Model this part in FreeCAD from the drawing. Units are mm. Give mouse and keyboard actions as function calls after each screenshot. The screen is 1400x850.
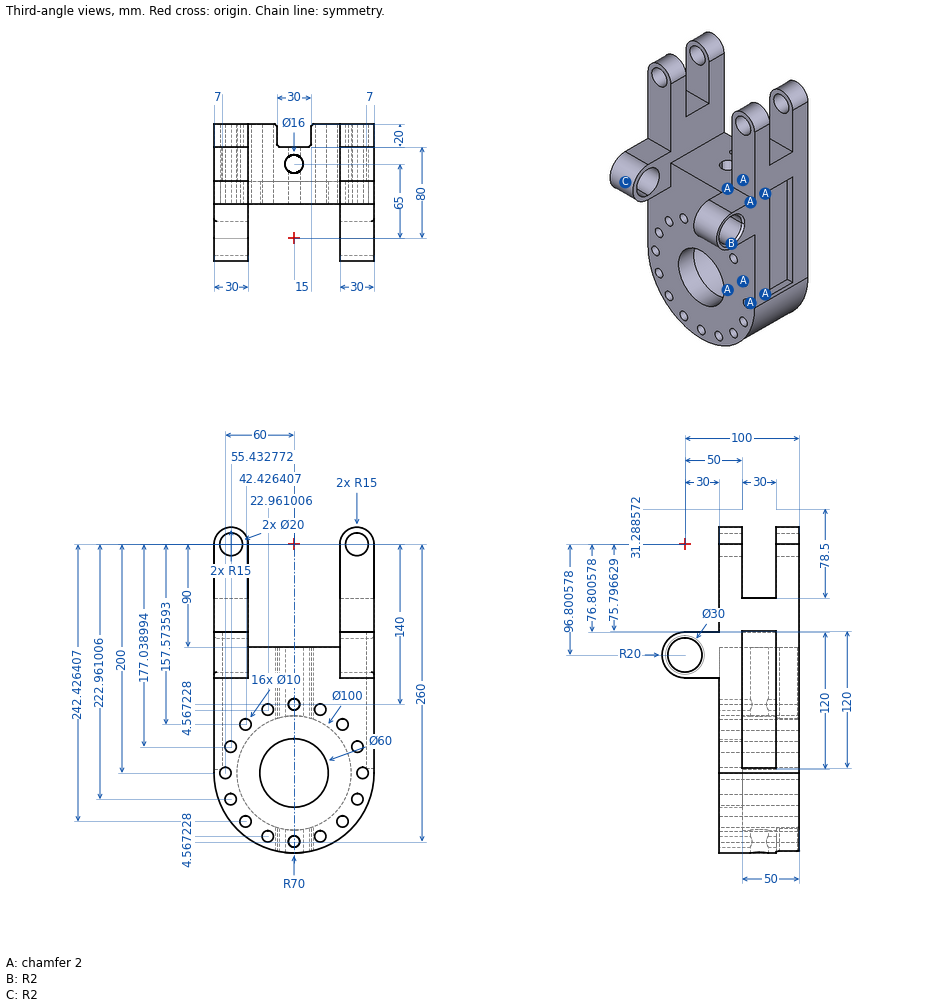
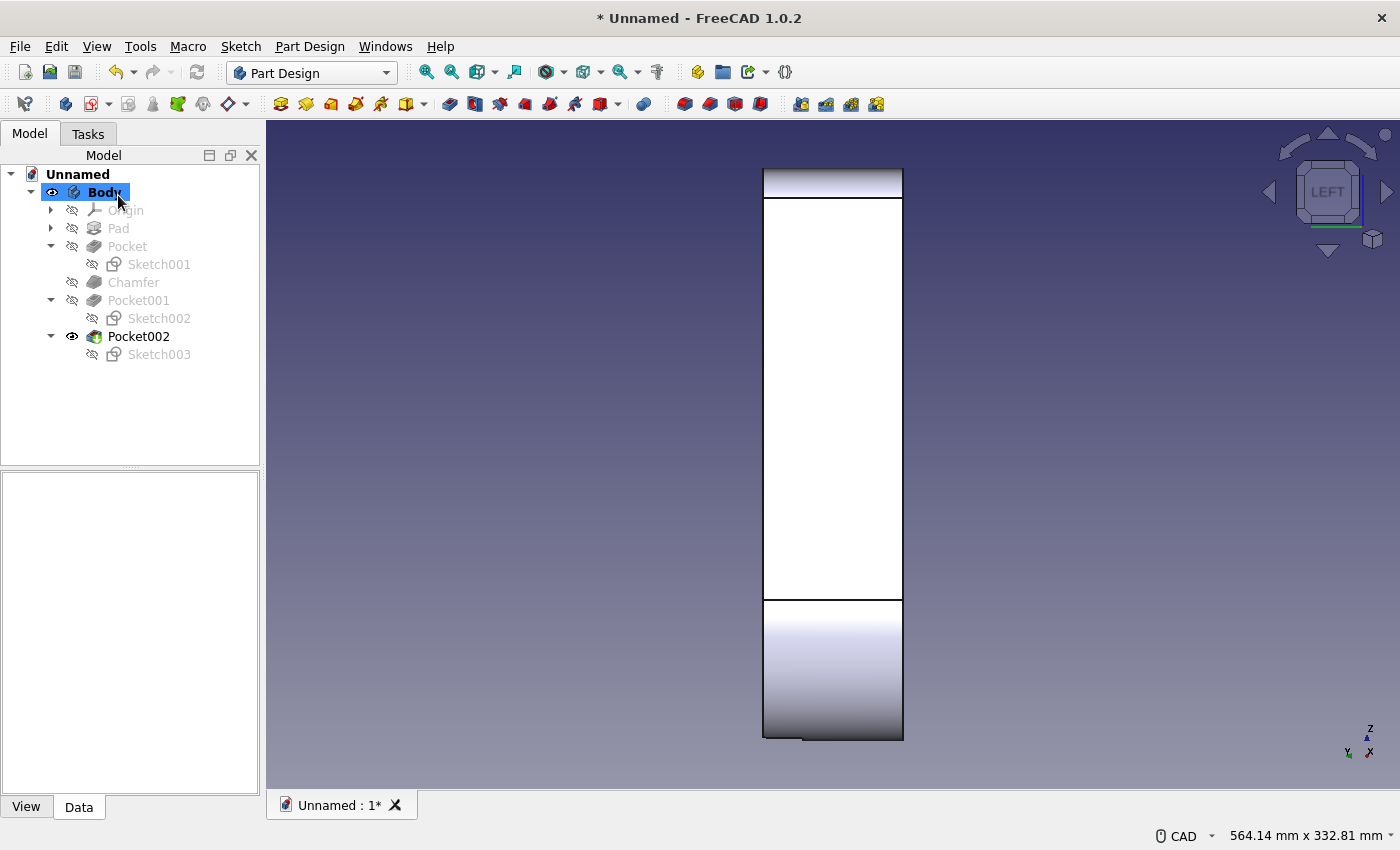
click(833, 513)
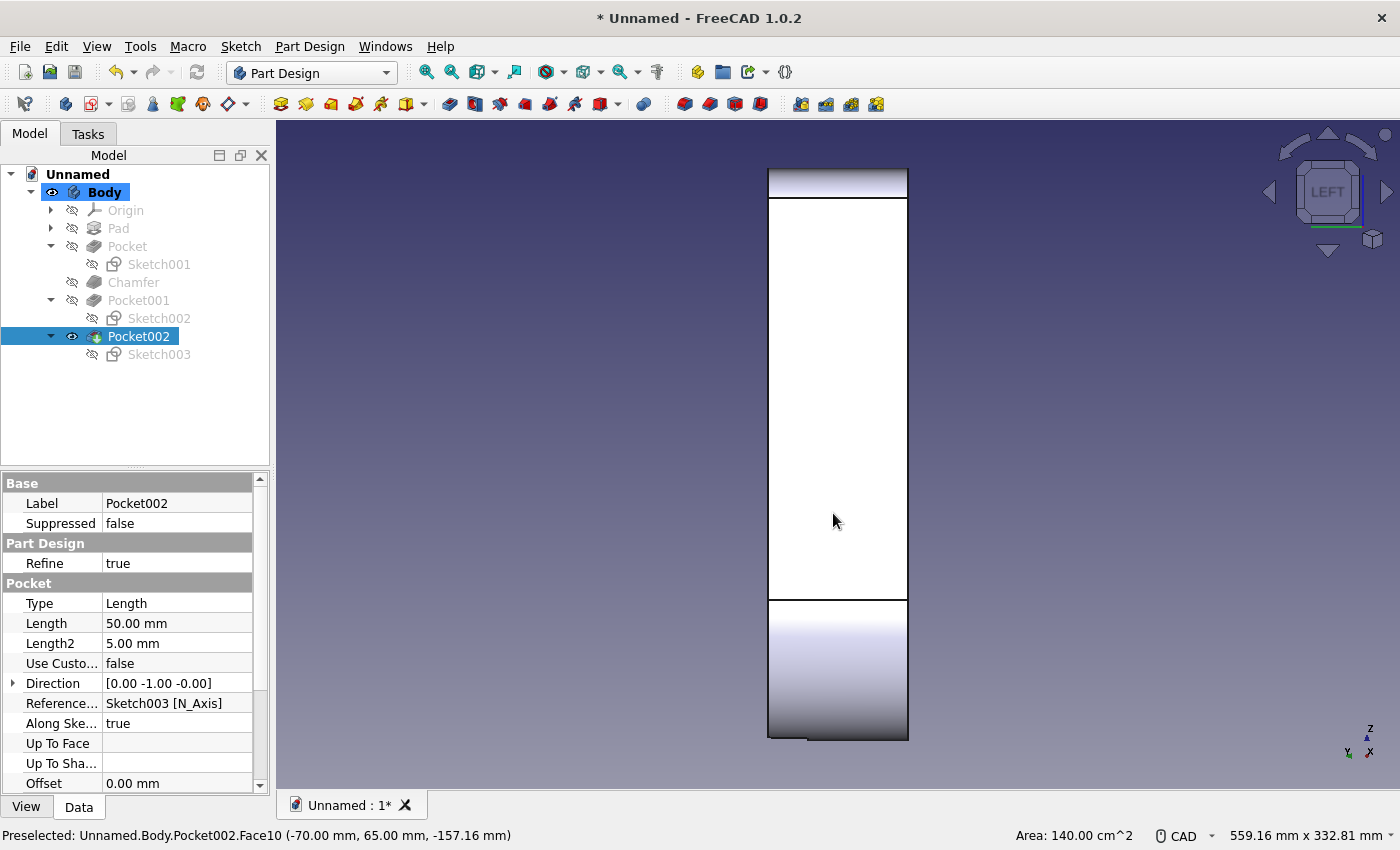
click(90, 104)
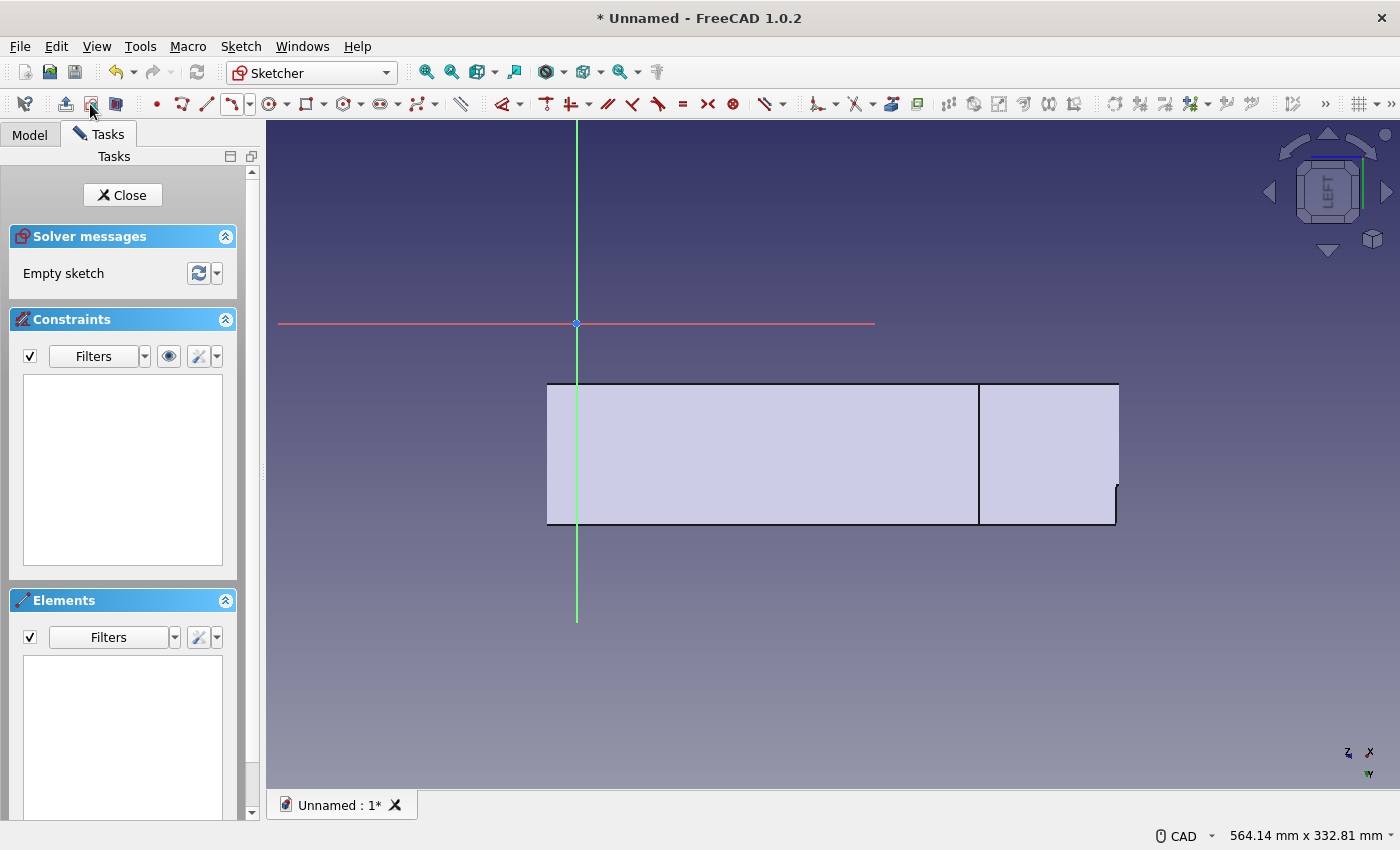
scroll(493, 375, up, 5)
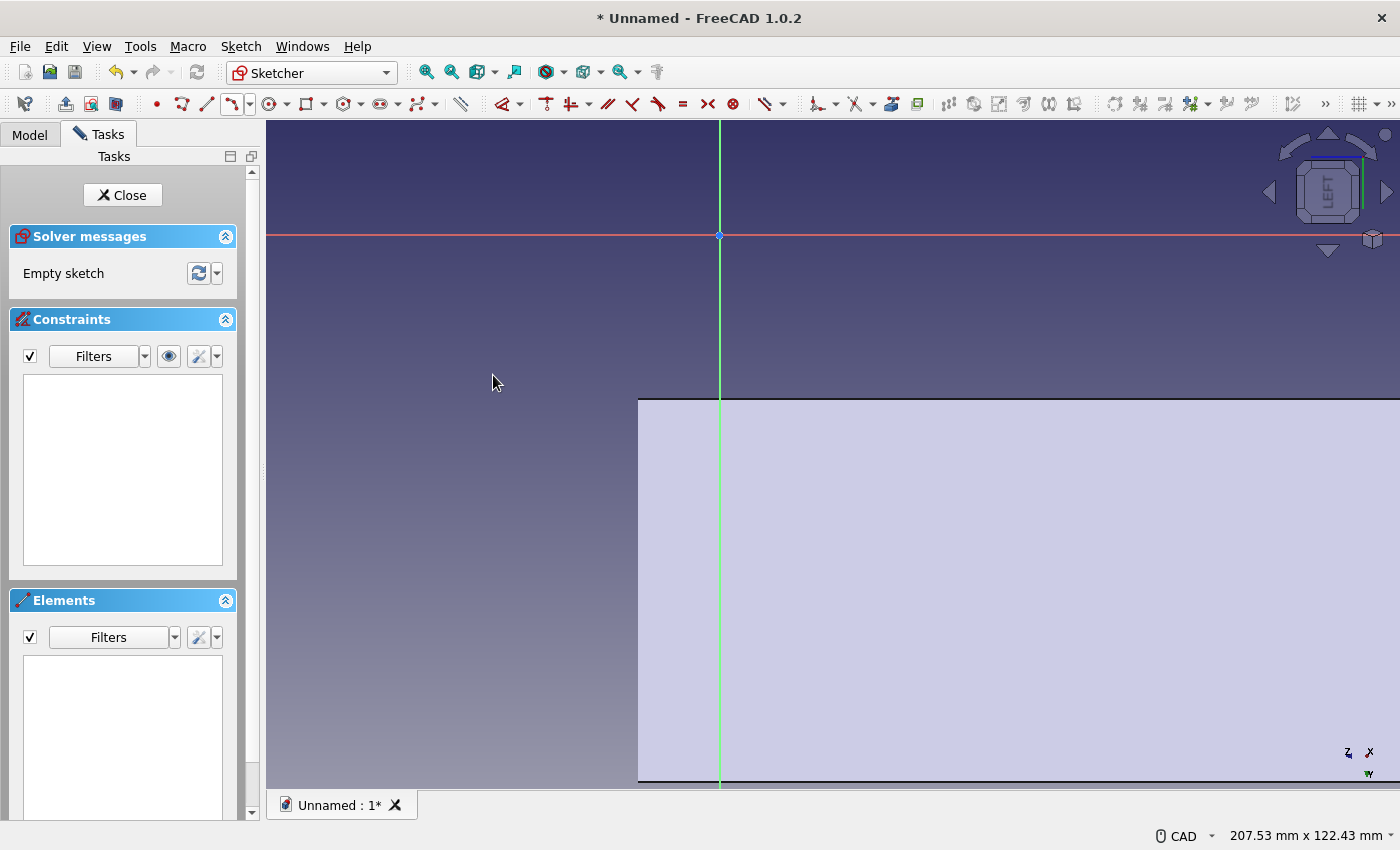
click(306, 104)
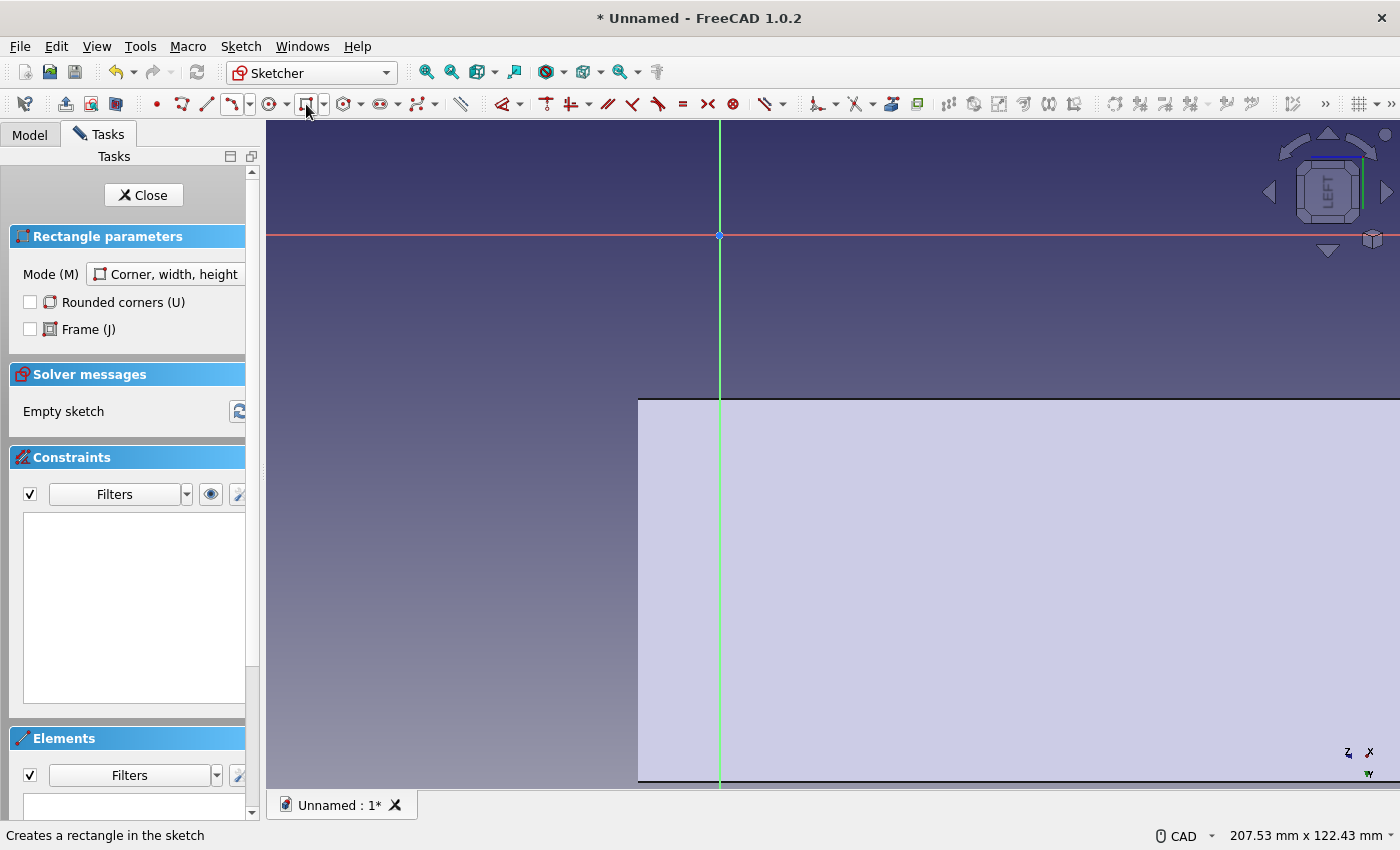
click(549, 508)
click(978, 672)
key(Escape)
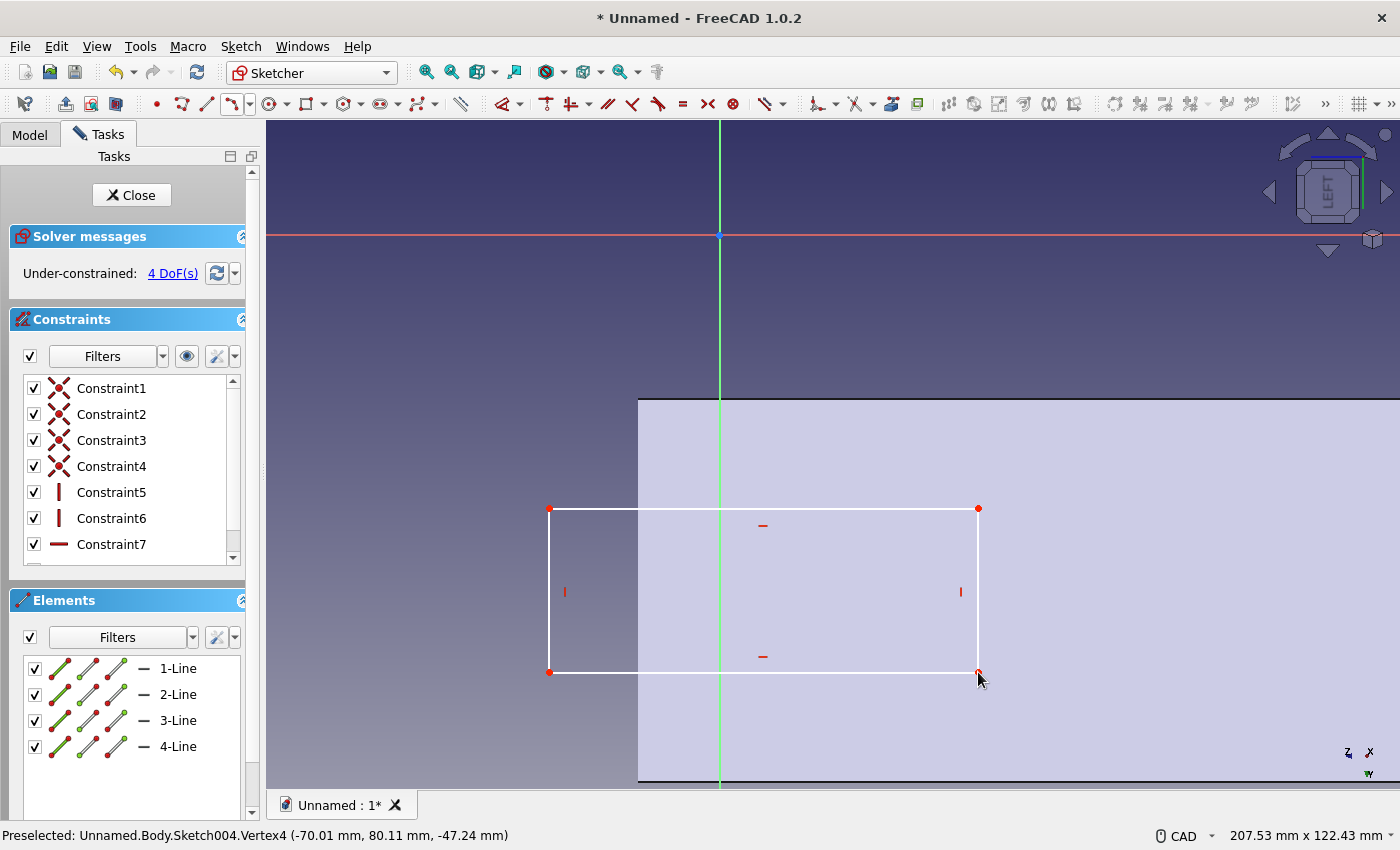
key(d)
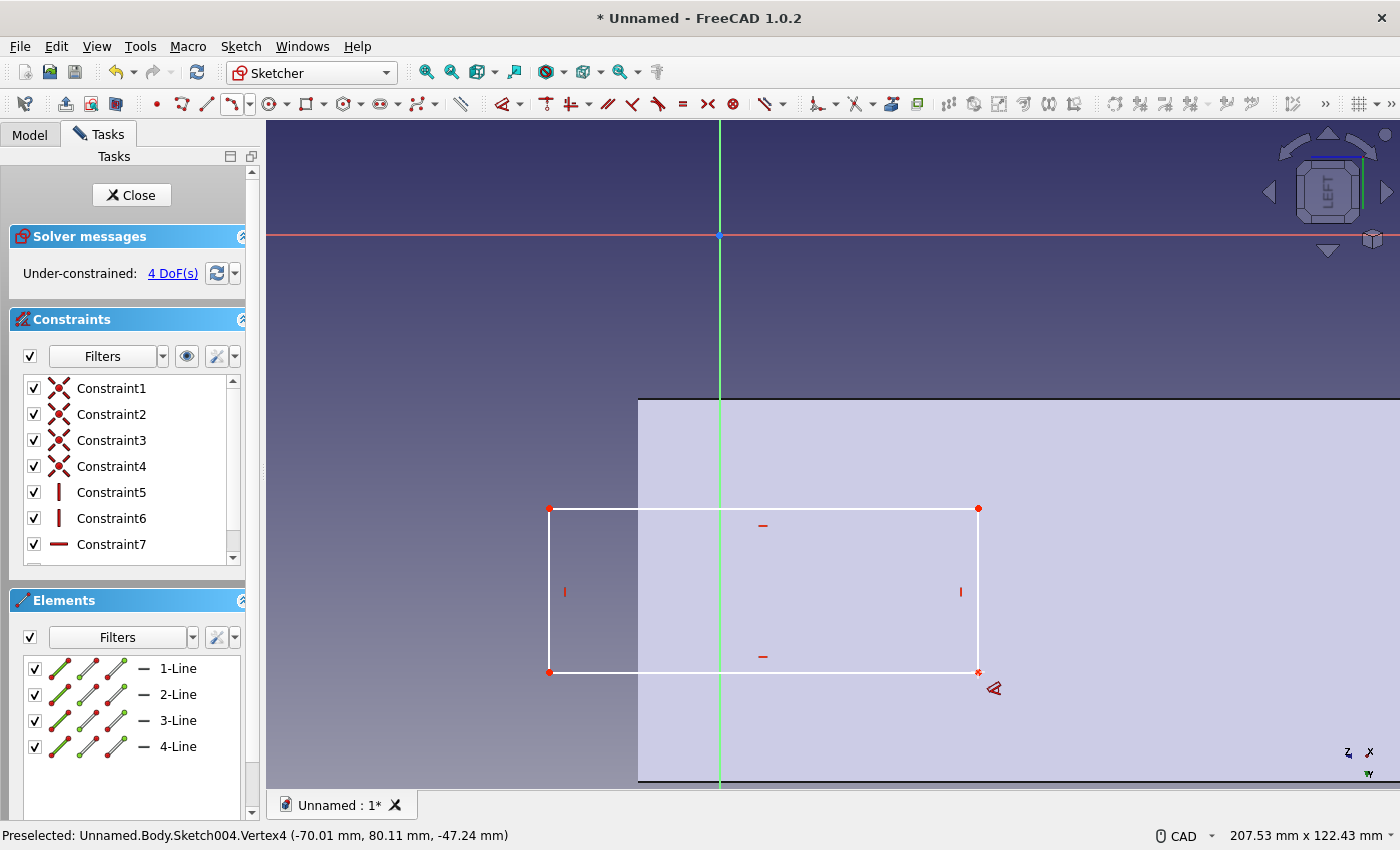
click(549, 558)
click(515, 591)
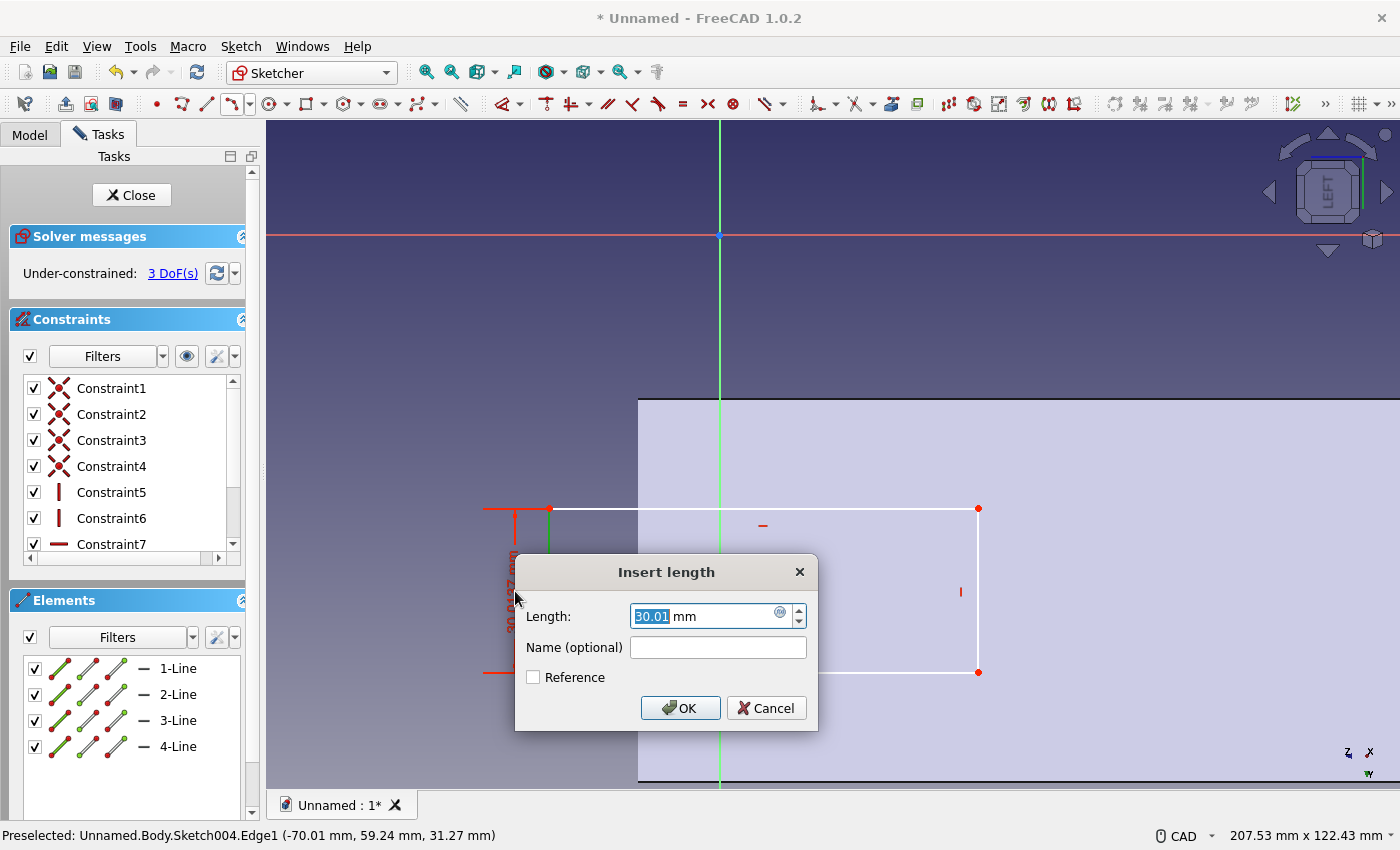
text(30)
key(Return)